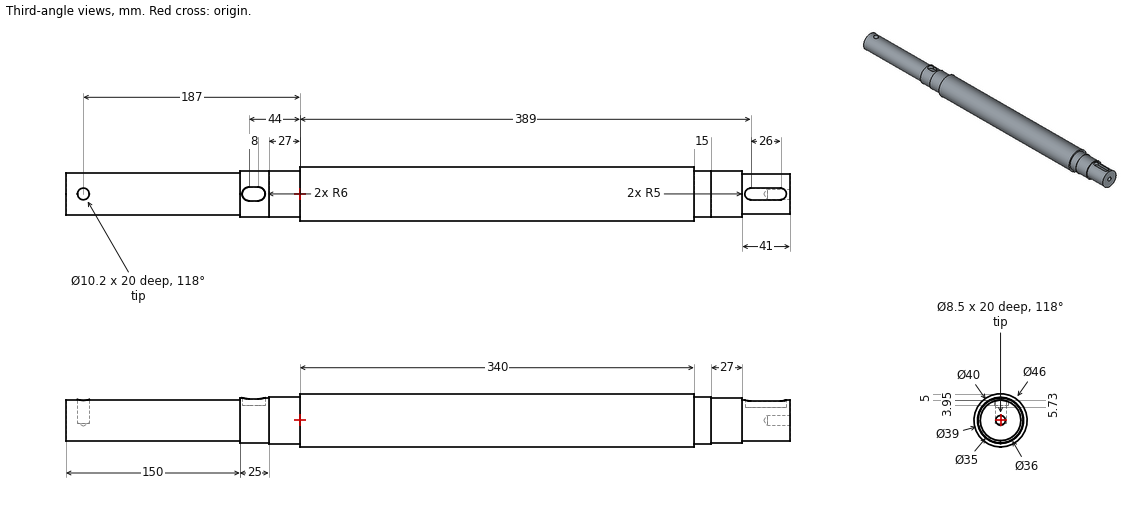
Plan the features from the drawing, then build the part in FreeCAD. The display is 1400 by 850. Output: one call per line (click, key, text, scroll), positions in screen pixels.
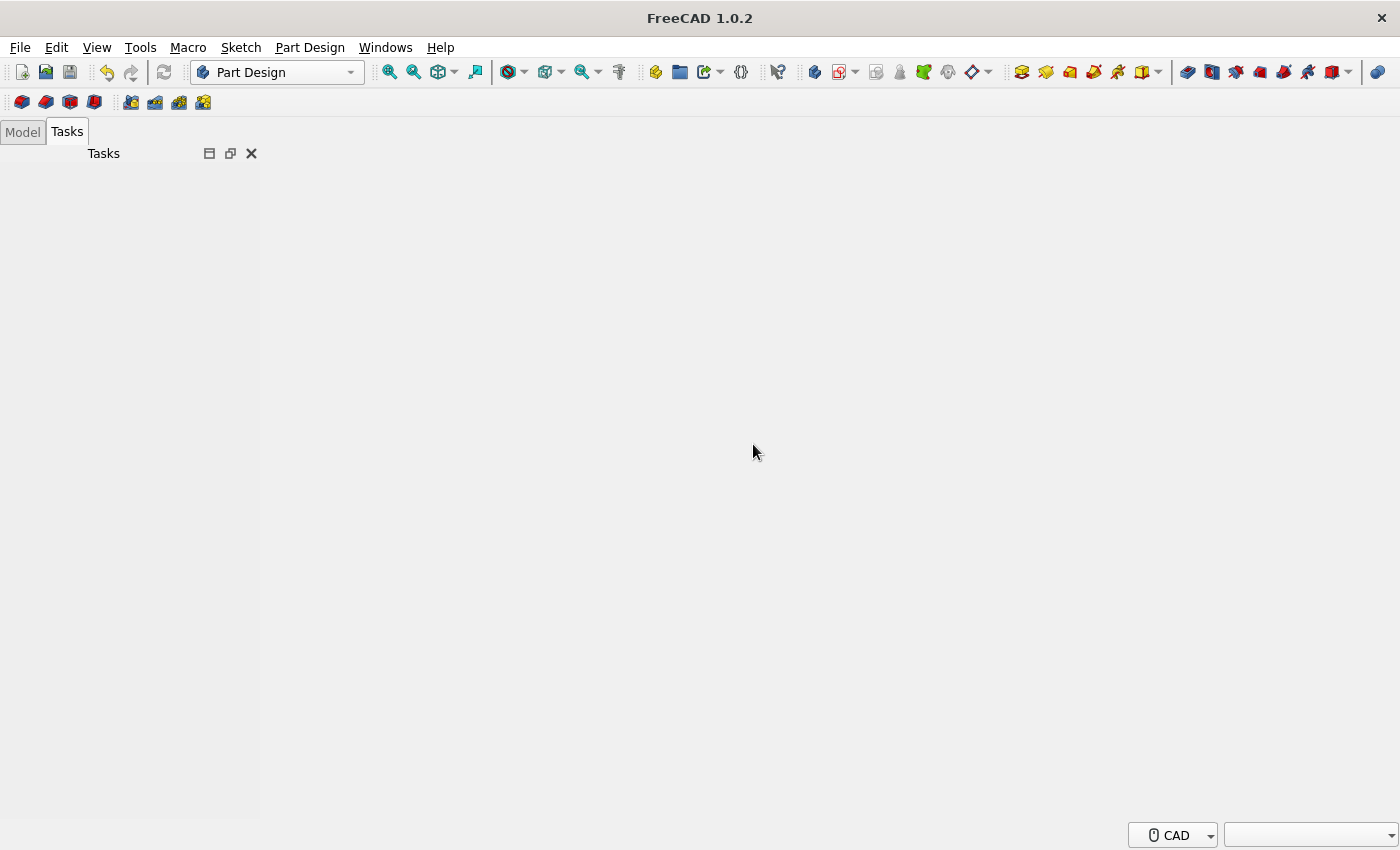
click(22, 72)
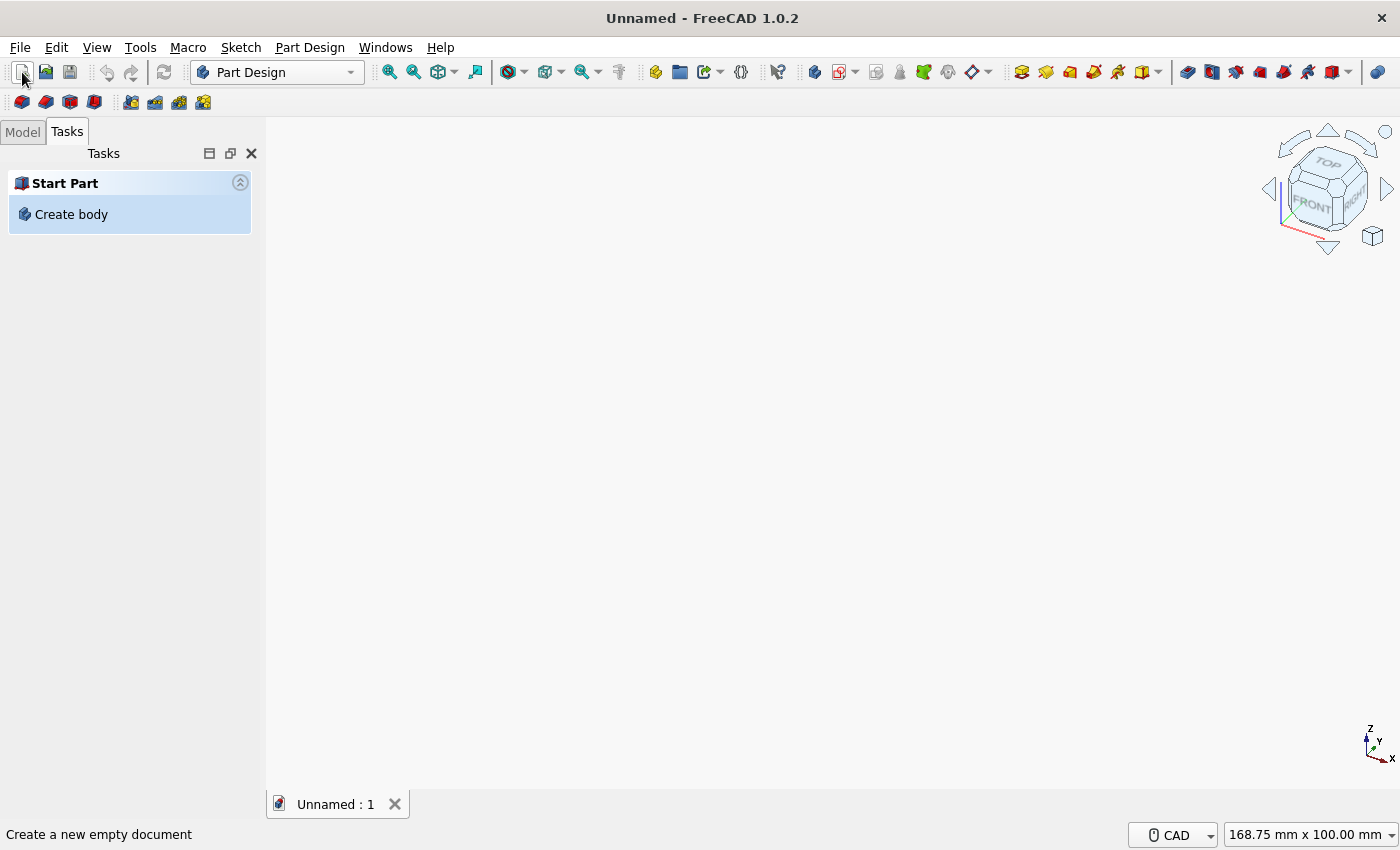
click(840, 72)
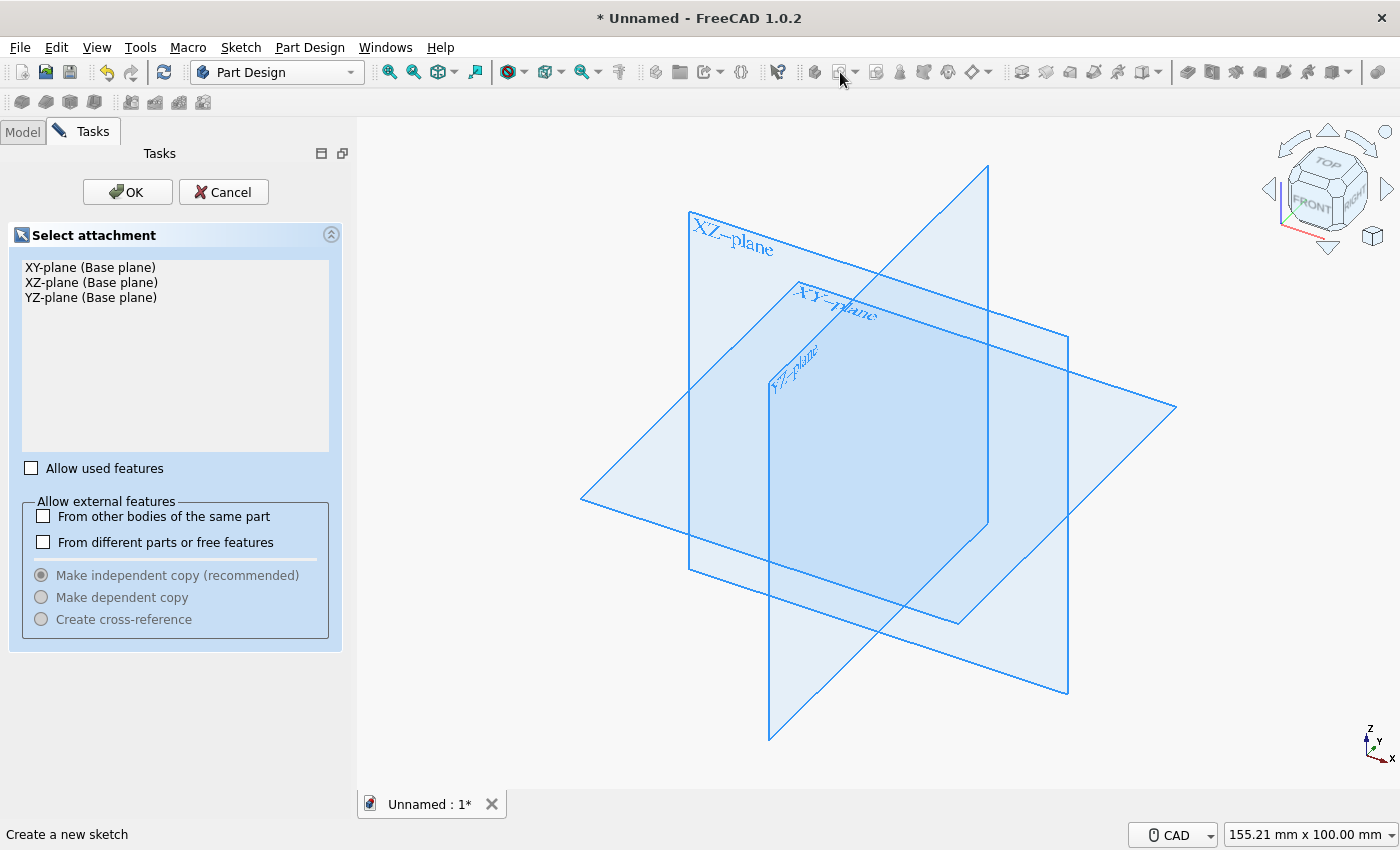
click(82, 298)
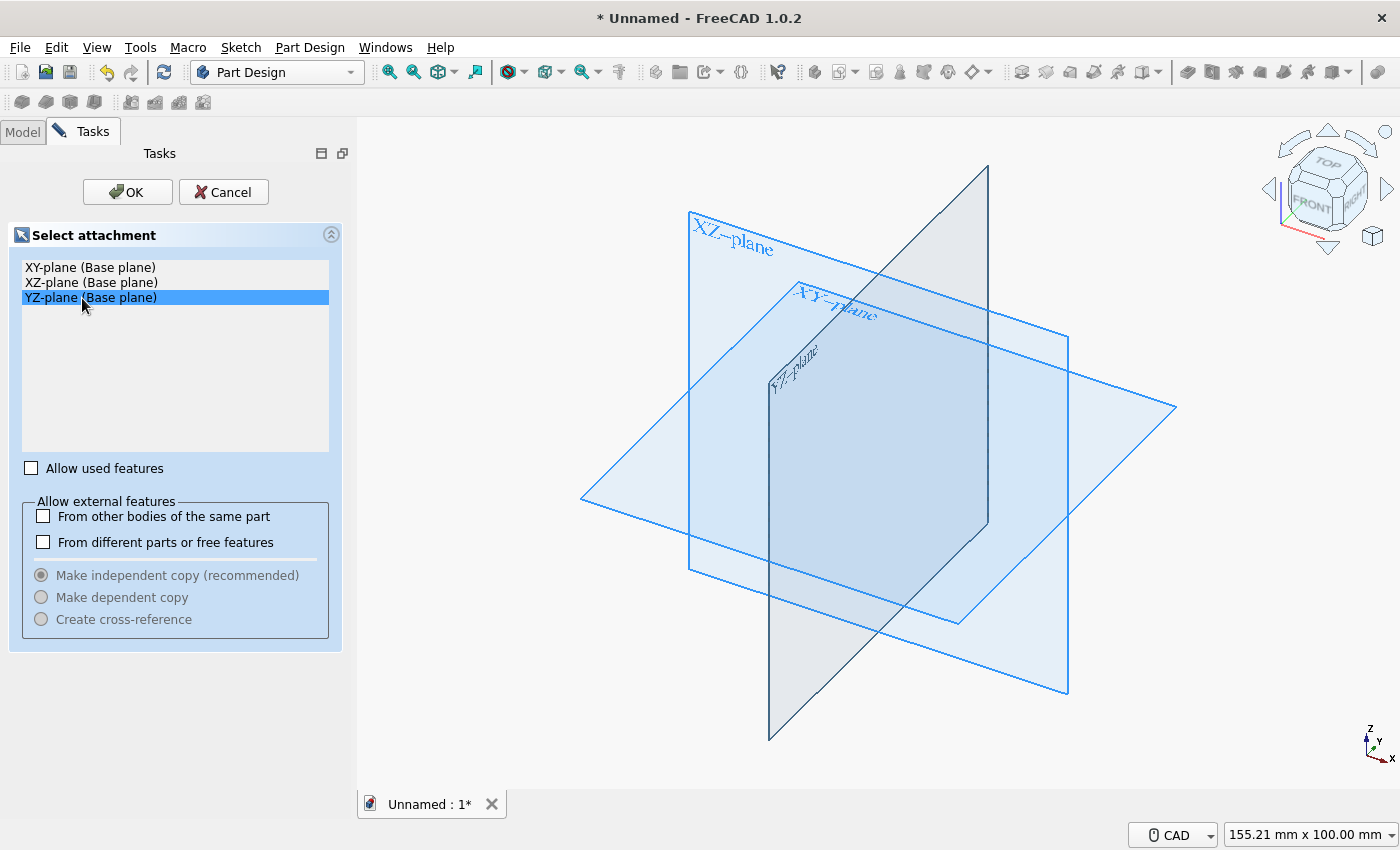
click(128, 192)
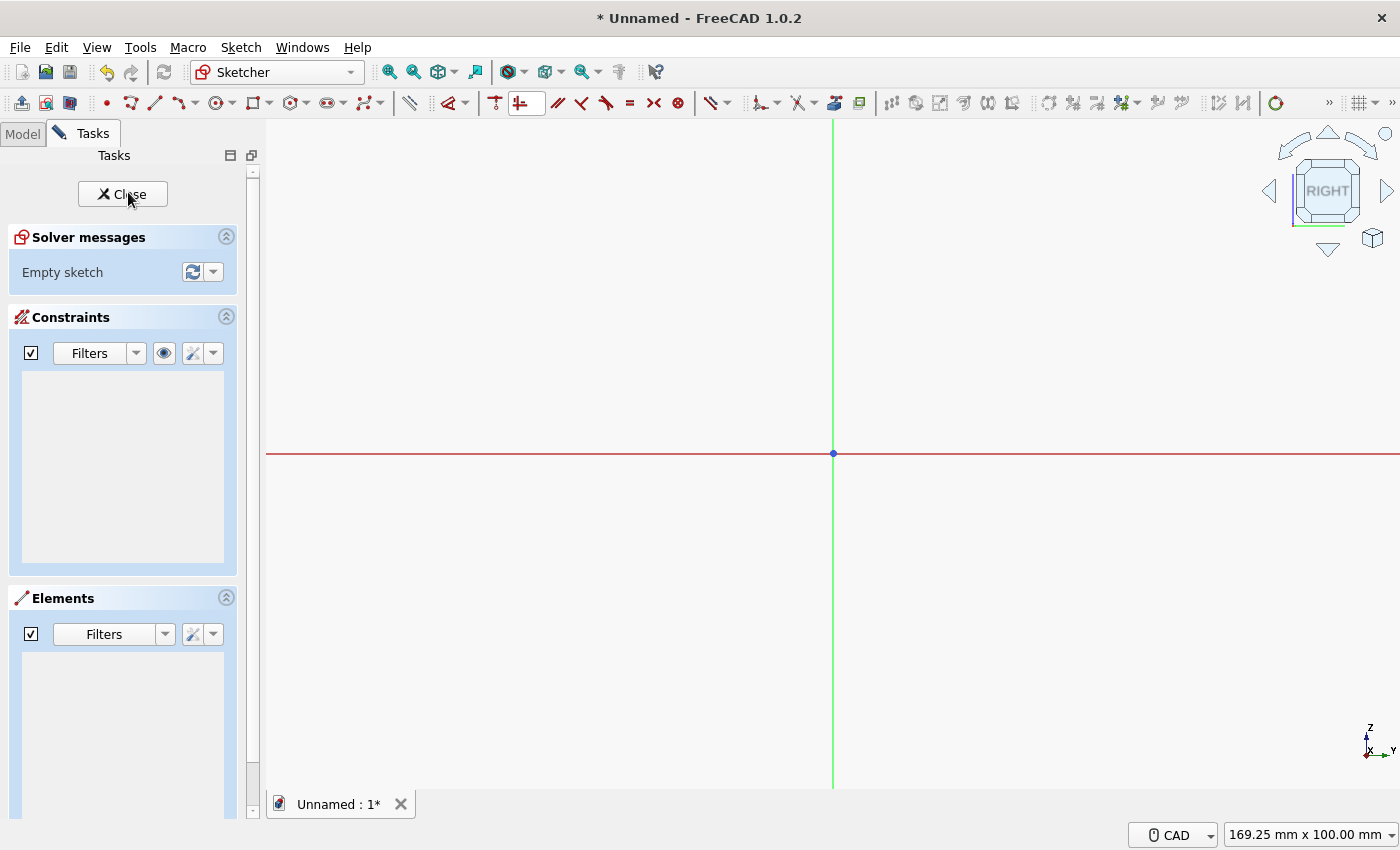
scroll(972, 454, up, 2)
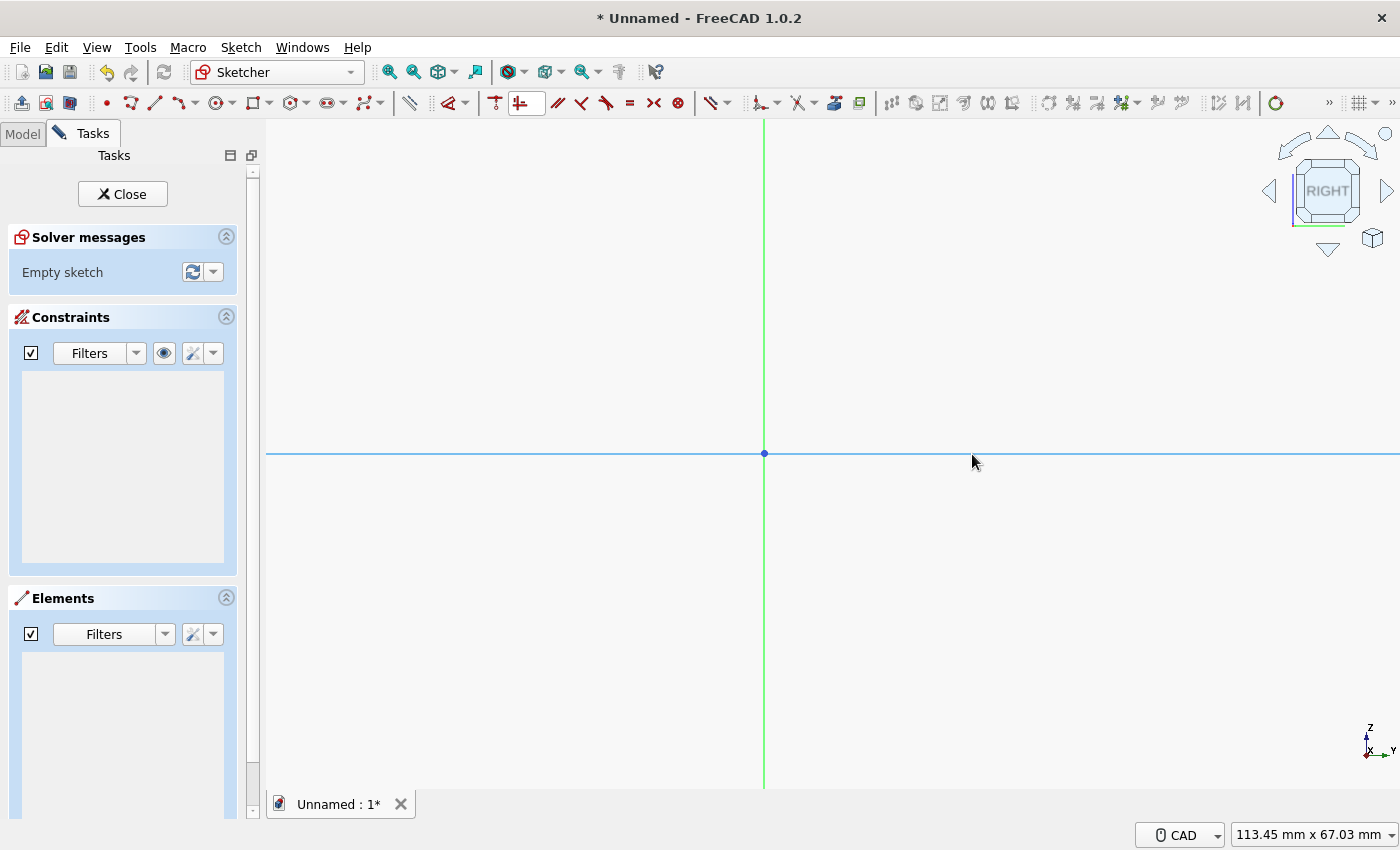
click(216, 104)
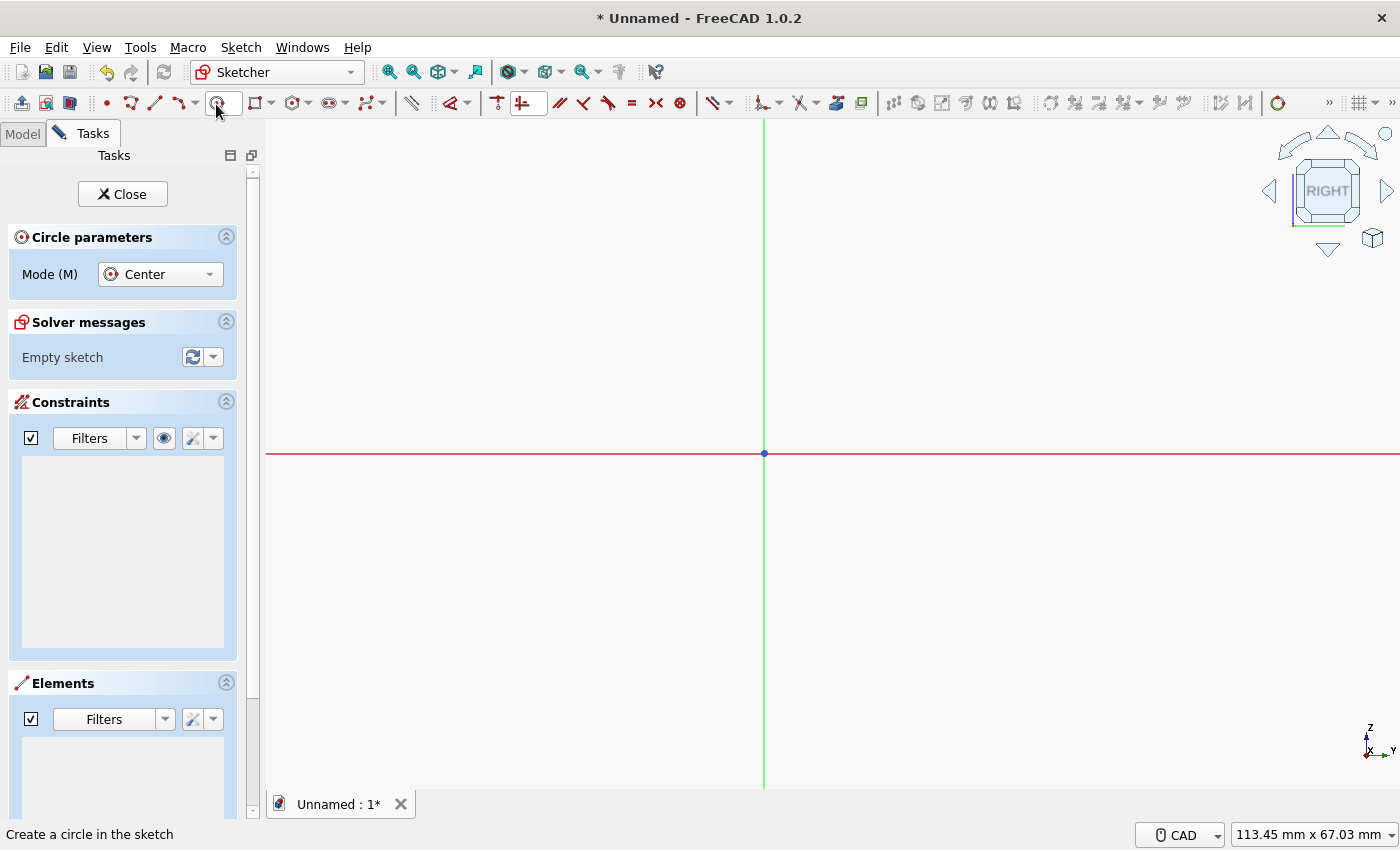
click(764, 454)
click(927, 291)
key(Escape)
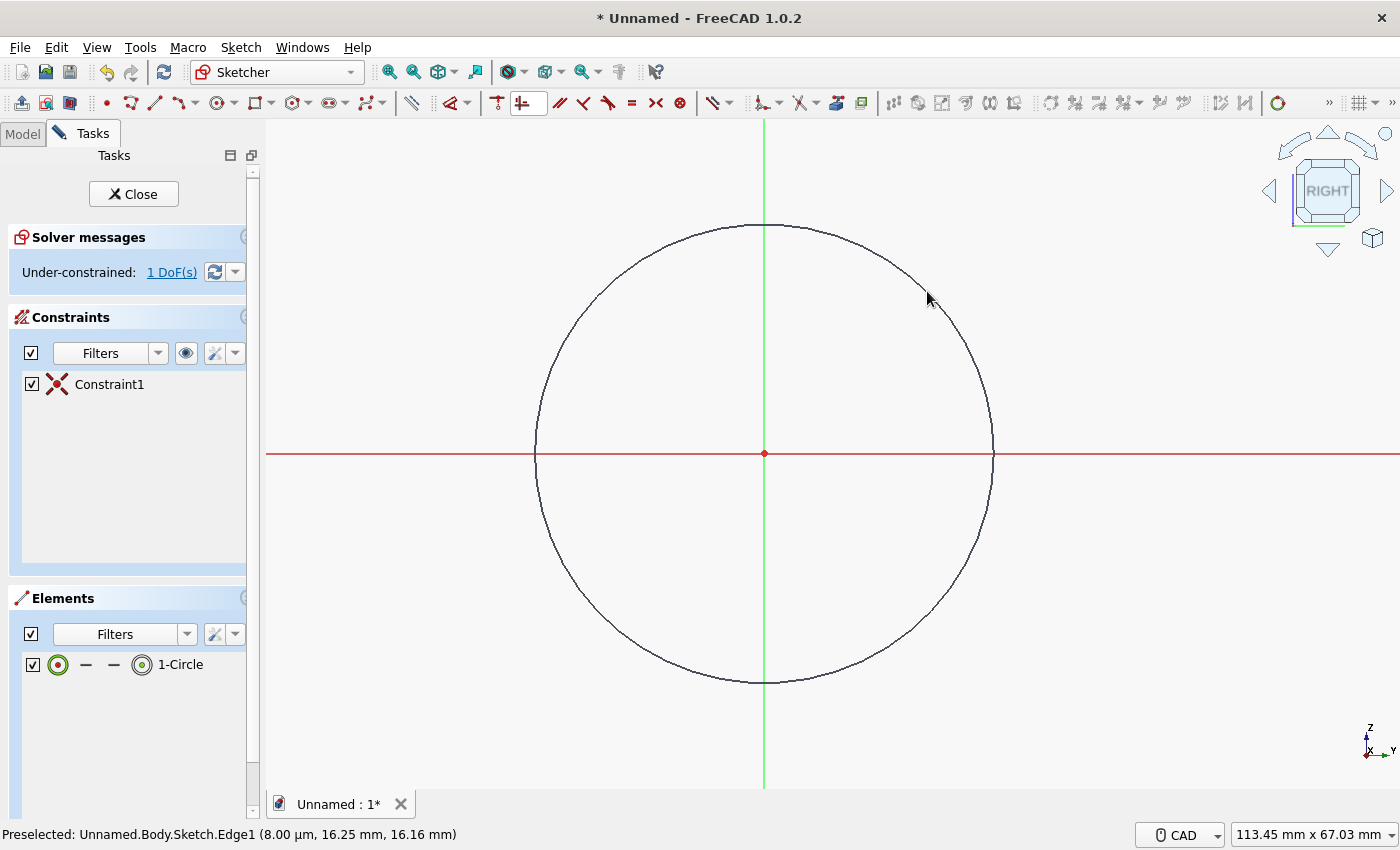
key(d)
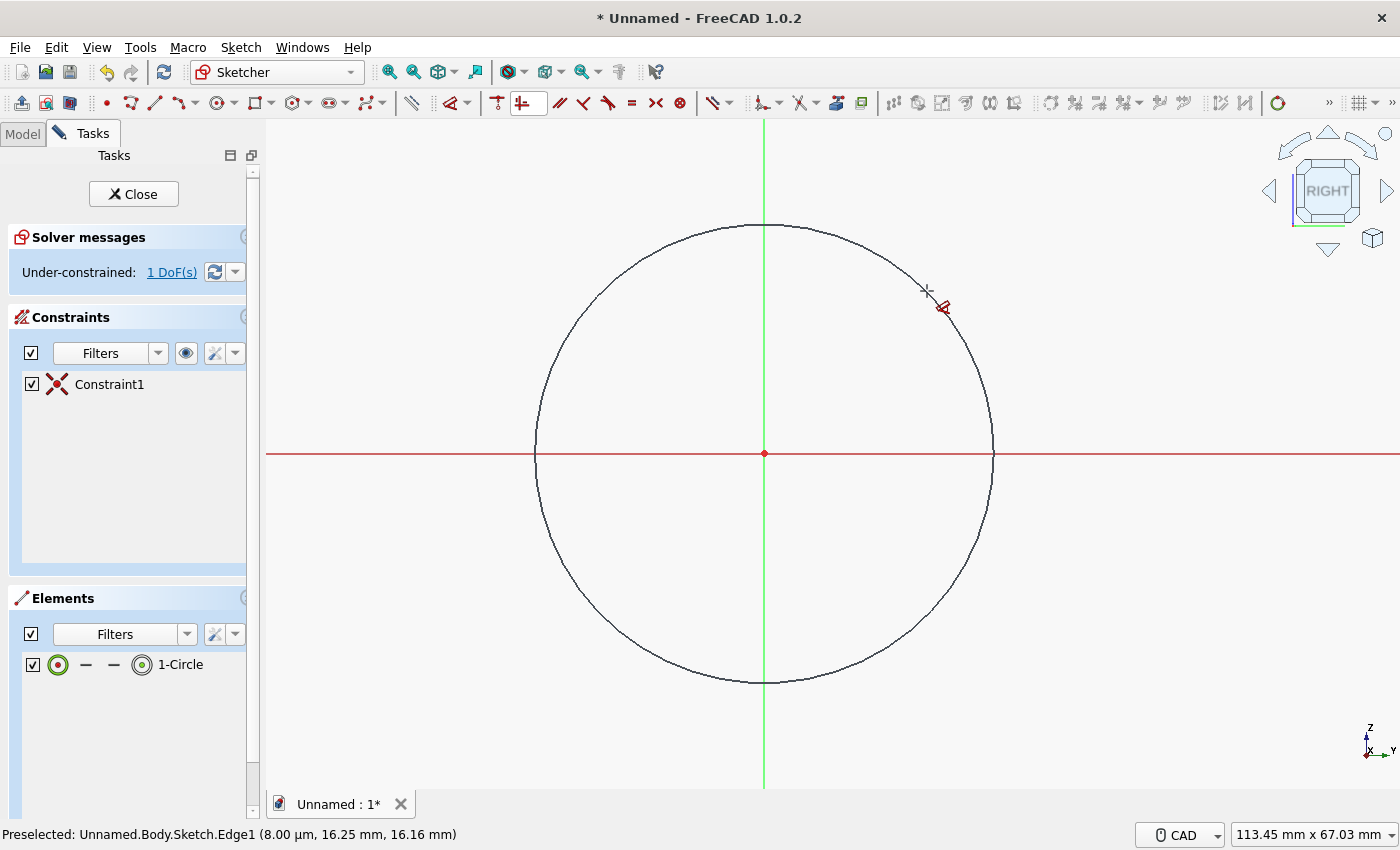
click(926, 291)
click(949, 268)